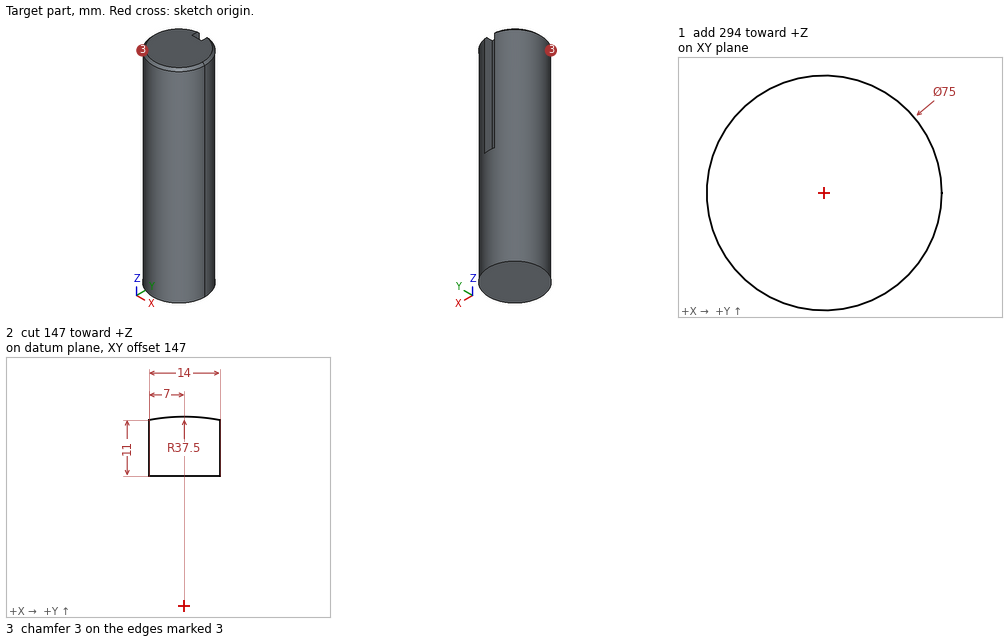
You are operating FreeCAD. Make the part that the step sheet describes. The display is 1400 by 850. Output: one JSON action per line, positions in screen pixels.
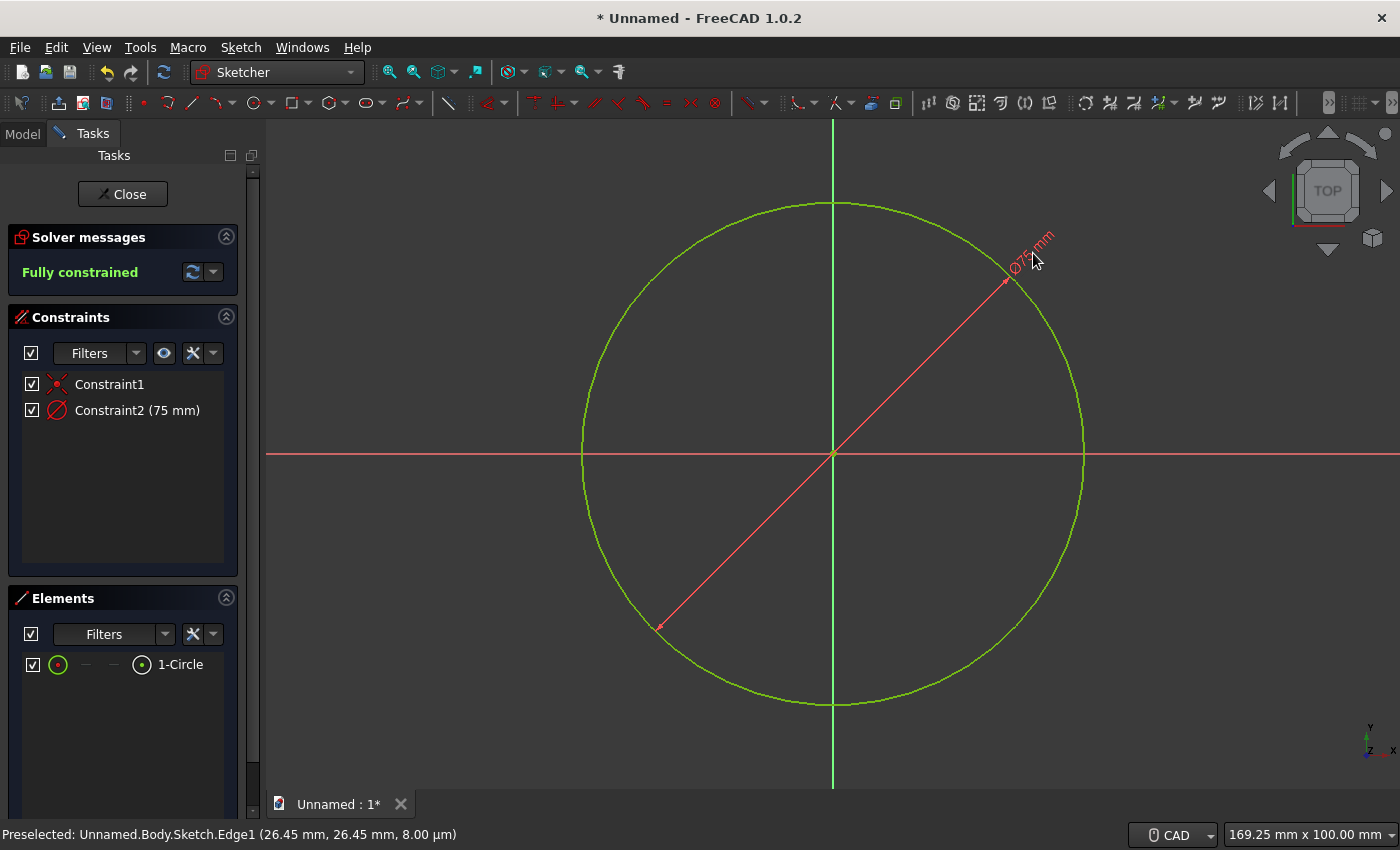
{"action": "left_click", "coordinate": [123, 194]}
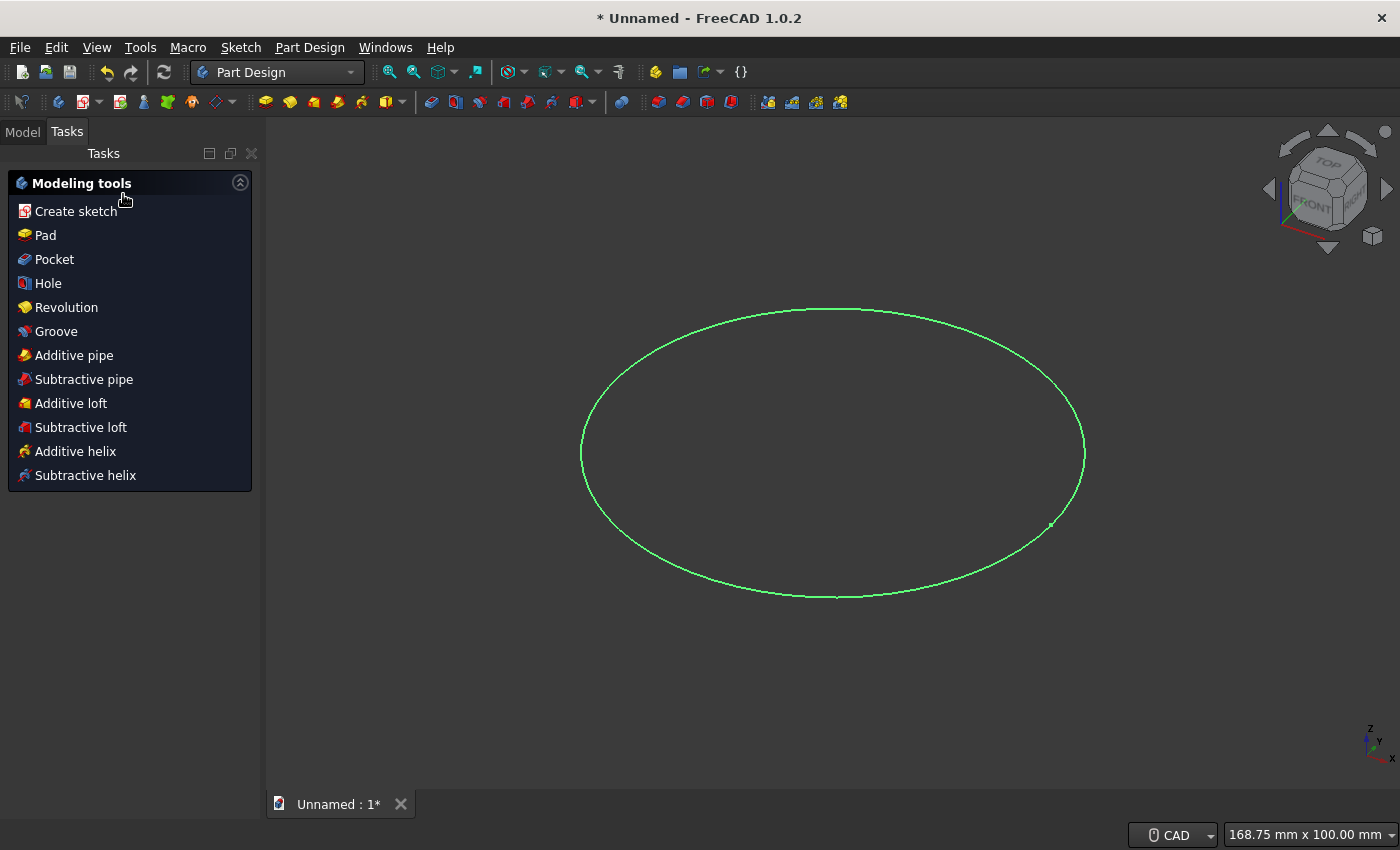
{"action": "left_click", "coordinate": [266, 102]}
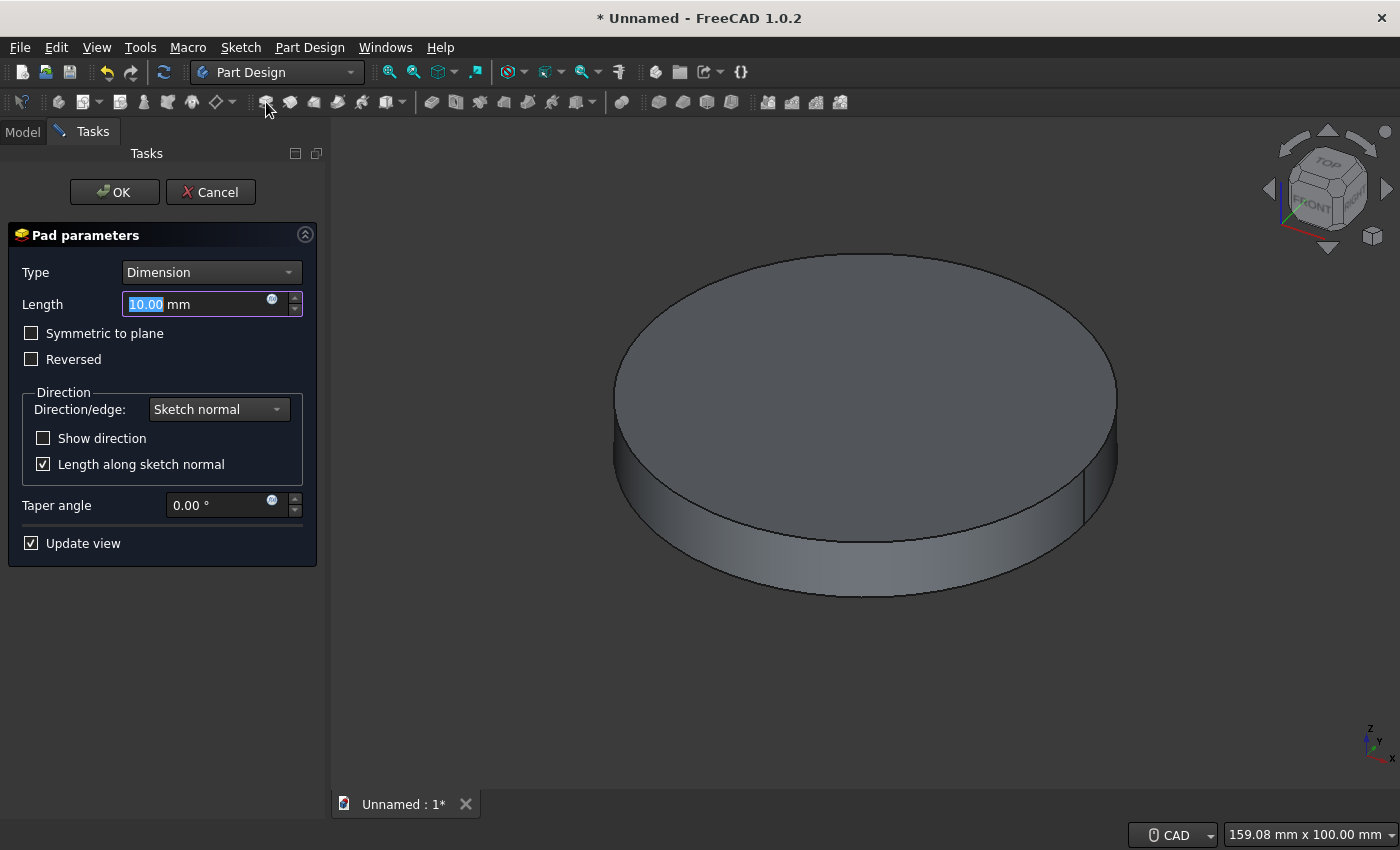
{"action": "type", "text": "294"}
{"action": "key", "text": "Tab"}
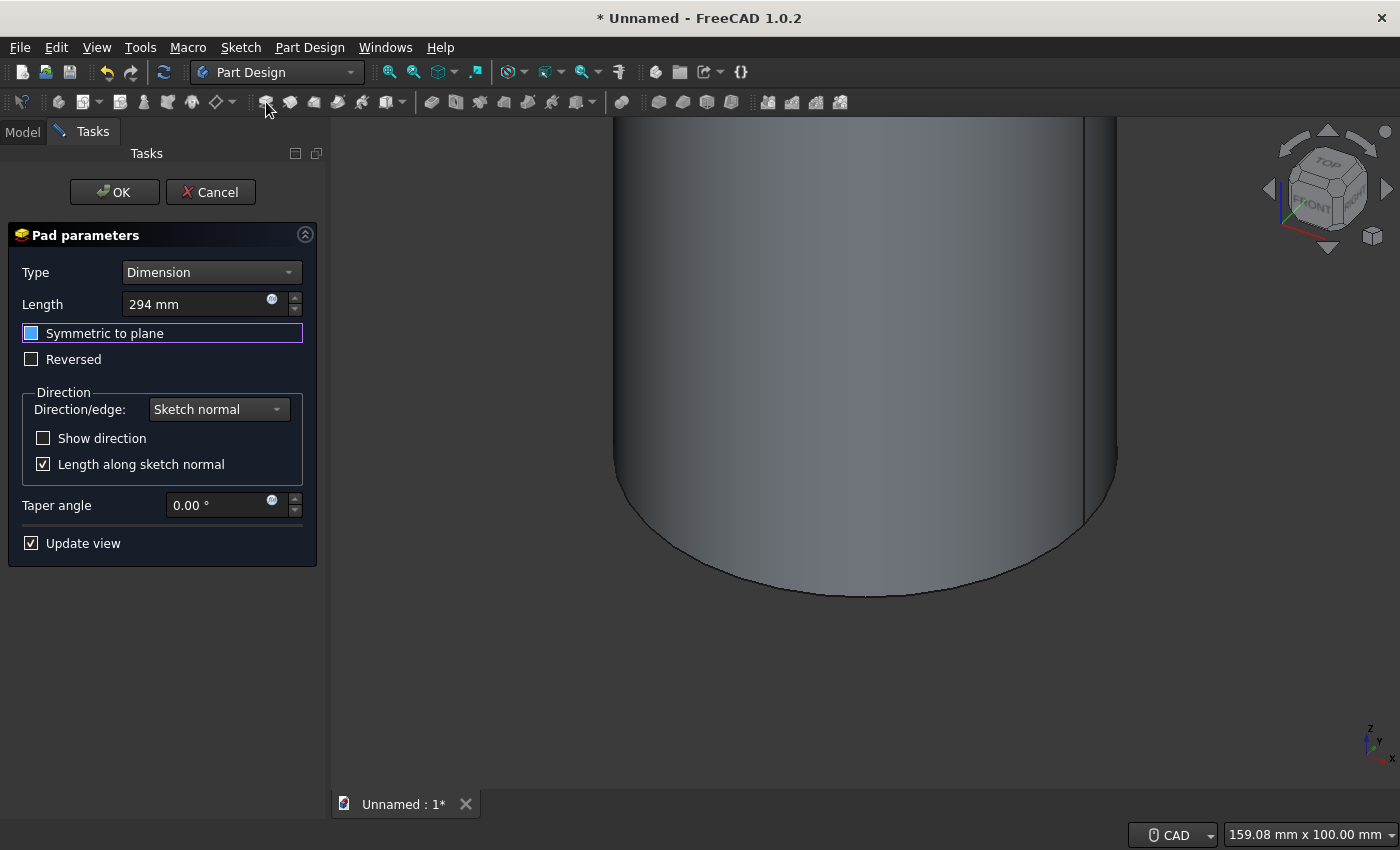
{"action": "left_click", "coordinate": [115, 192]}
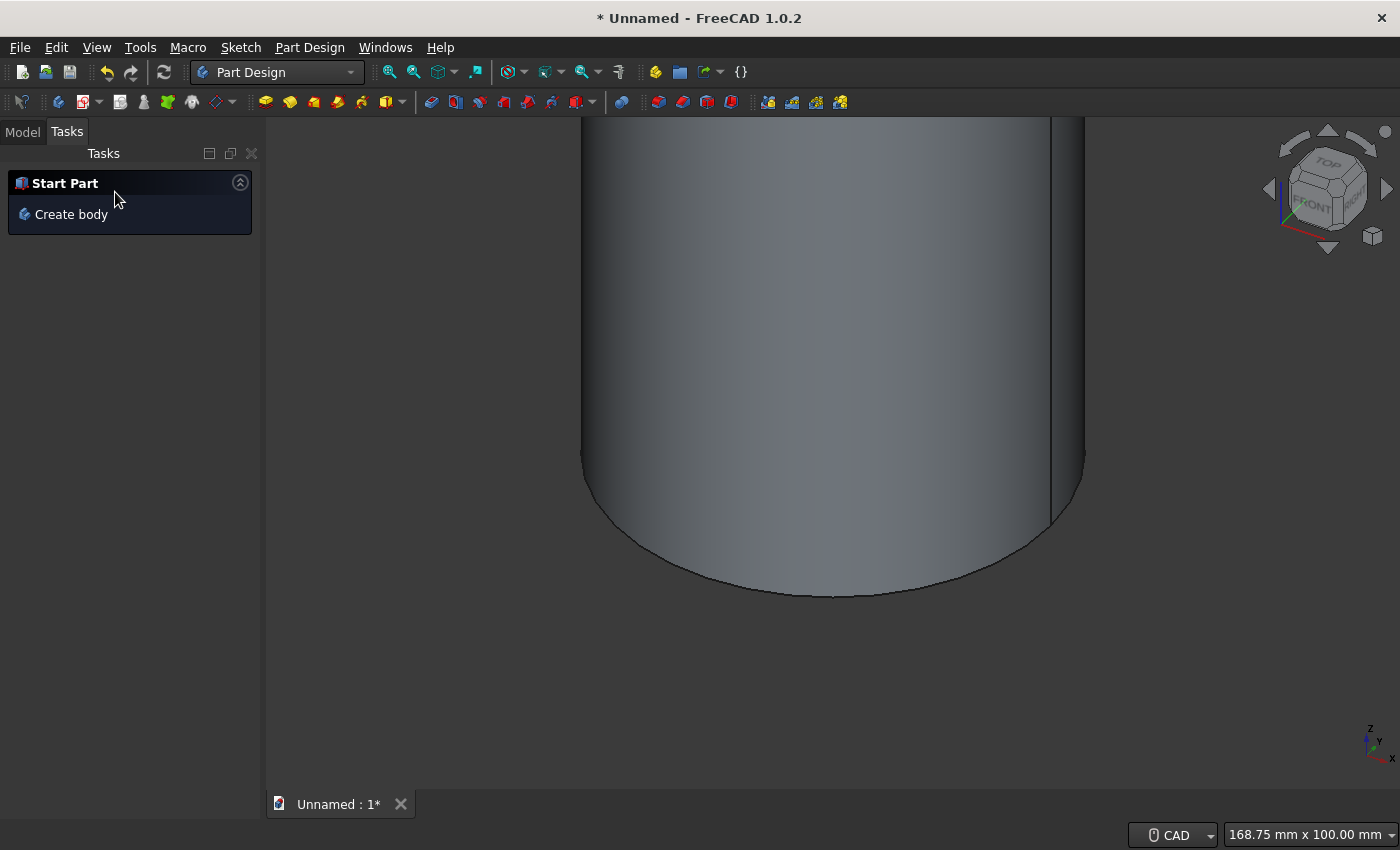
{"action": "left_click", "coordinate": [390, 72]}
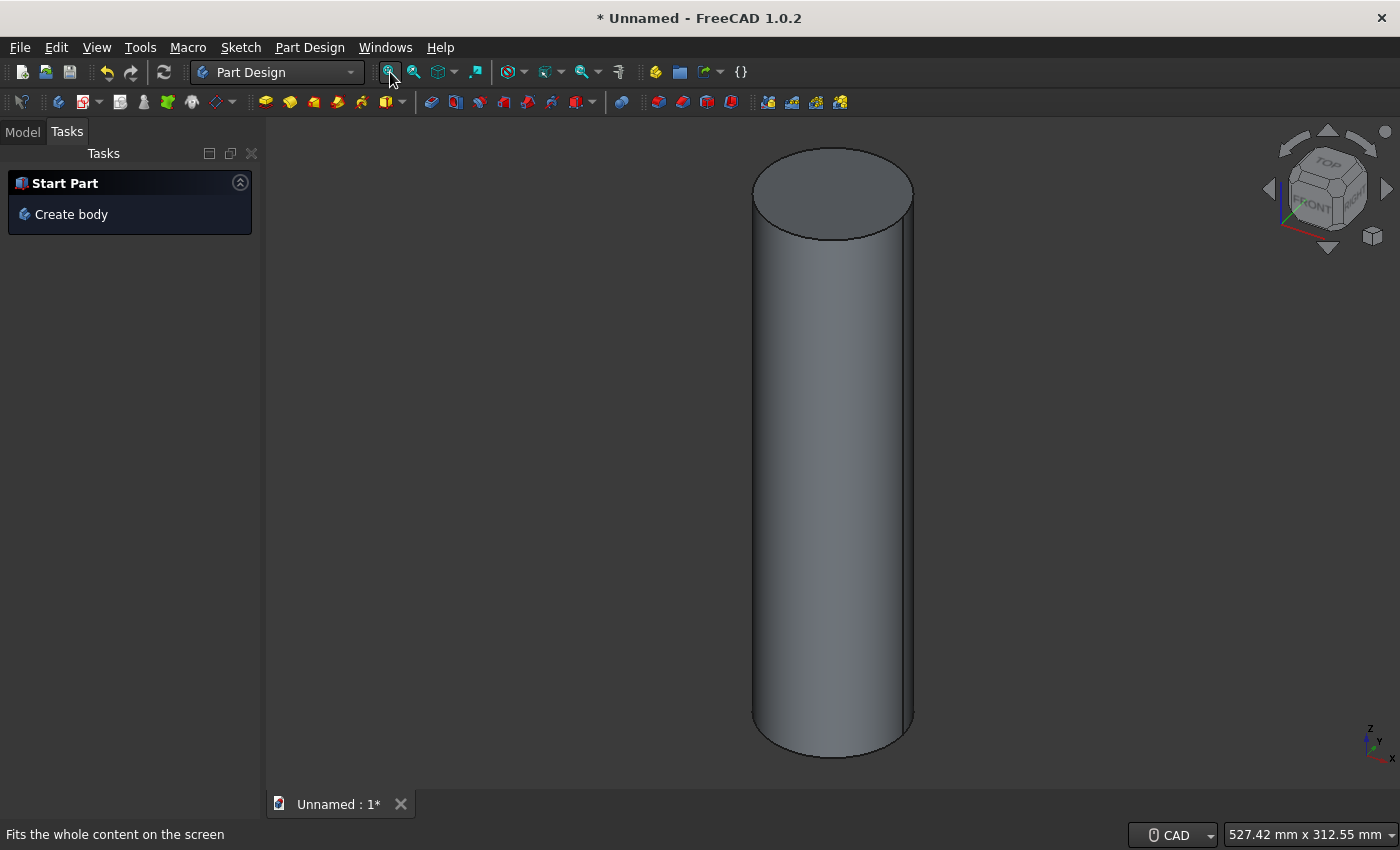
{"action": "left_click", "coordinate": [23, 131]}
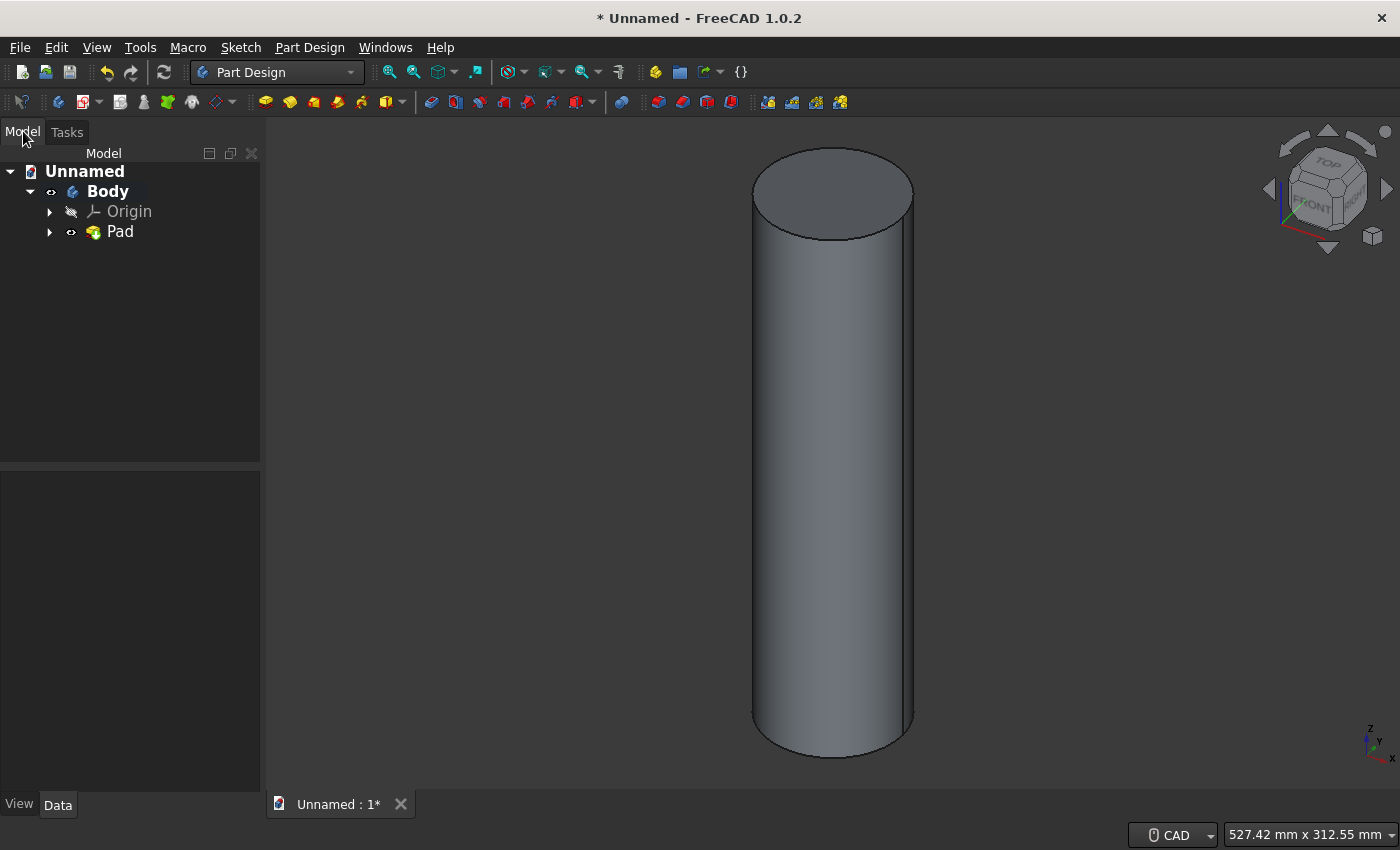
{"action": "left_click", "coordinate": [50, 212]}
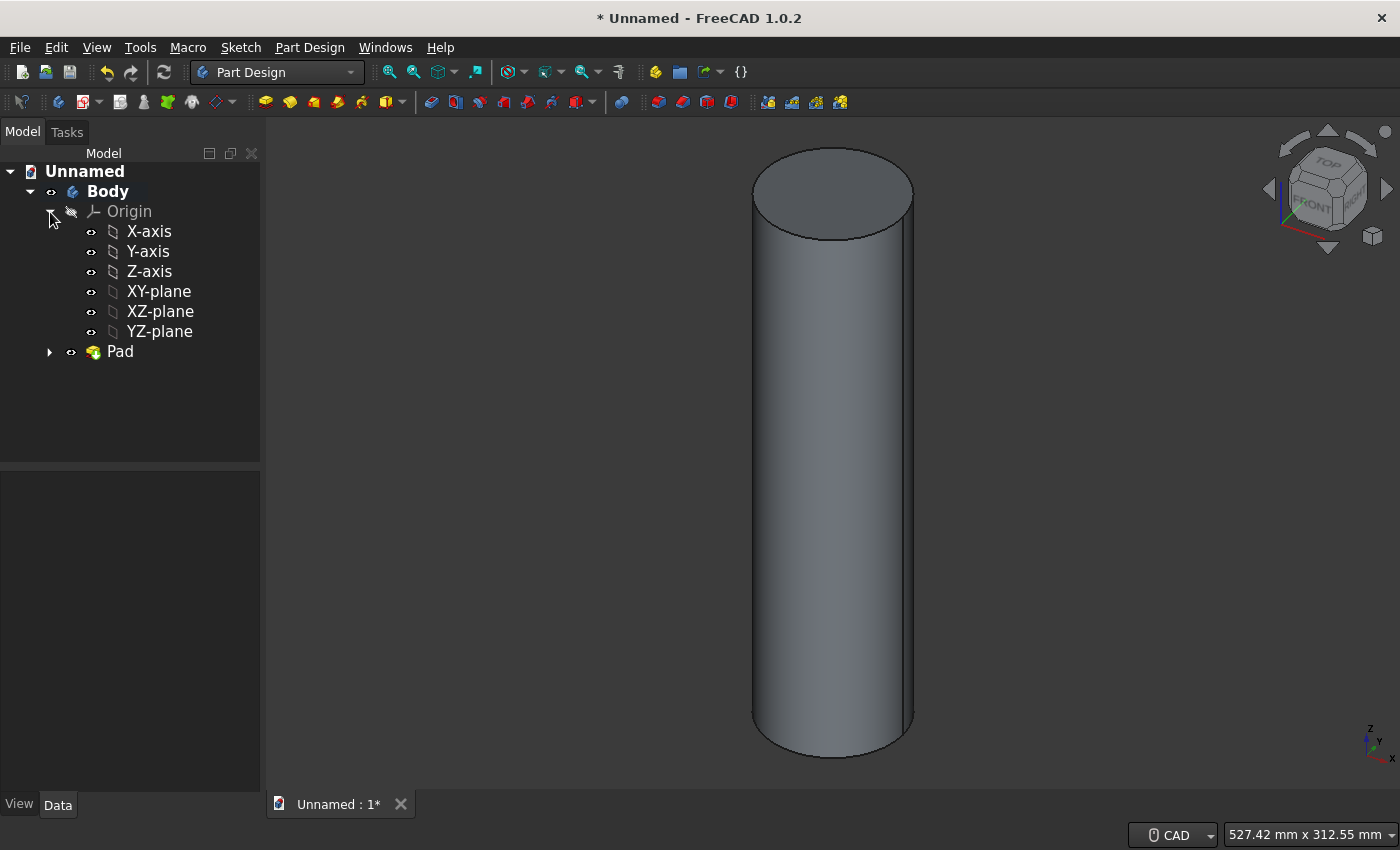
{"action": "left_click", "coordinate": [136, 292]}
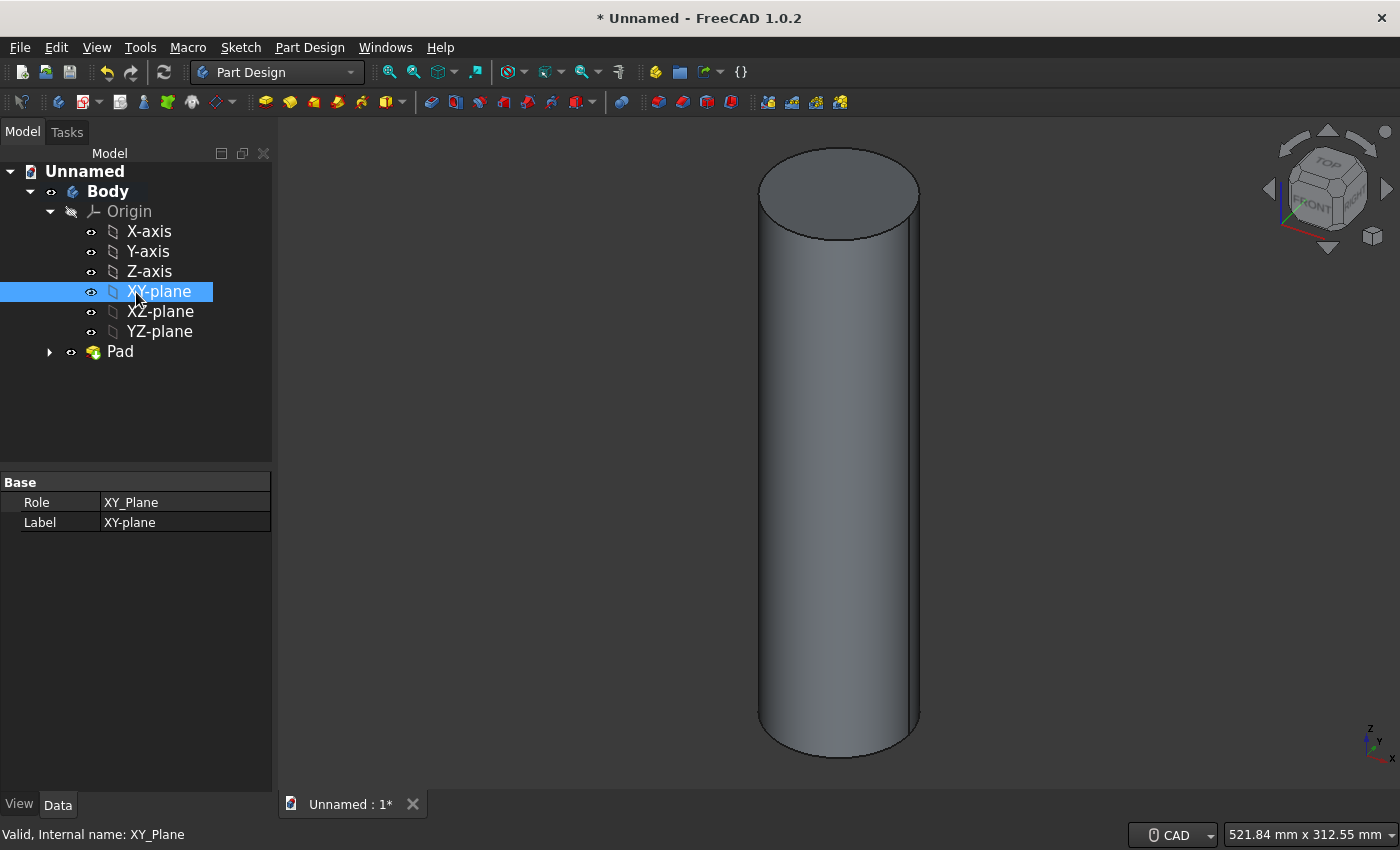
{"action": "left_click", "coordinate": [216, 102]}